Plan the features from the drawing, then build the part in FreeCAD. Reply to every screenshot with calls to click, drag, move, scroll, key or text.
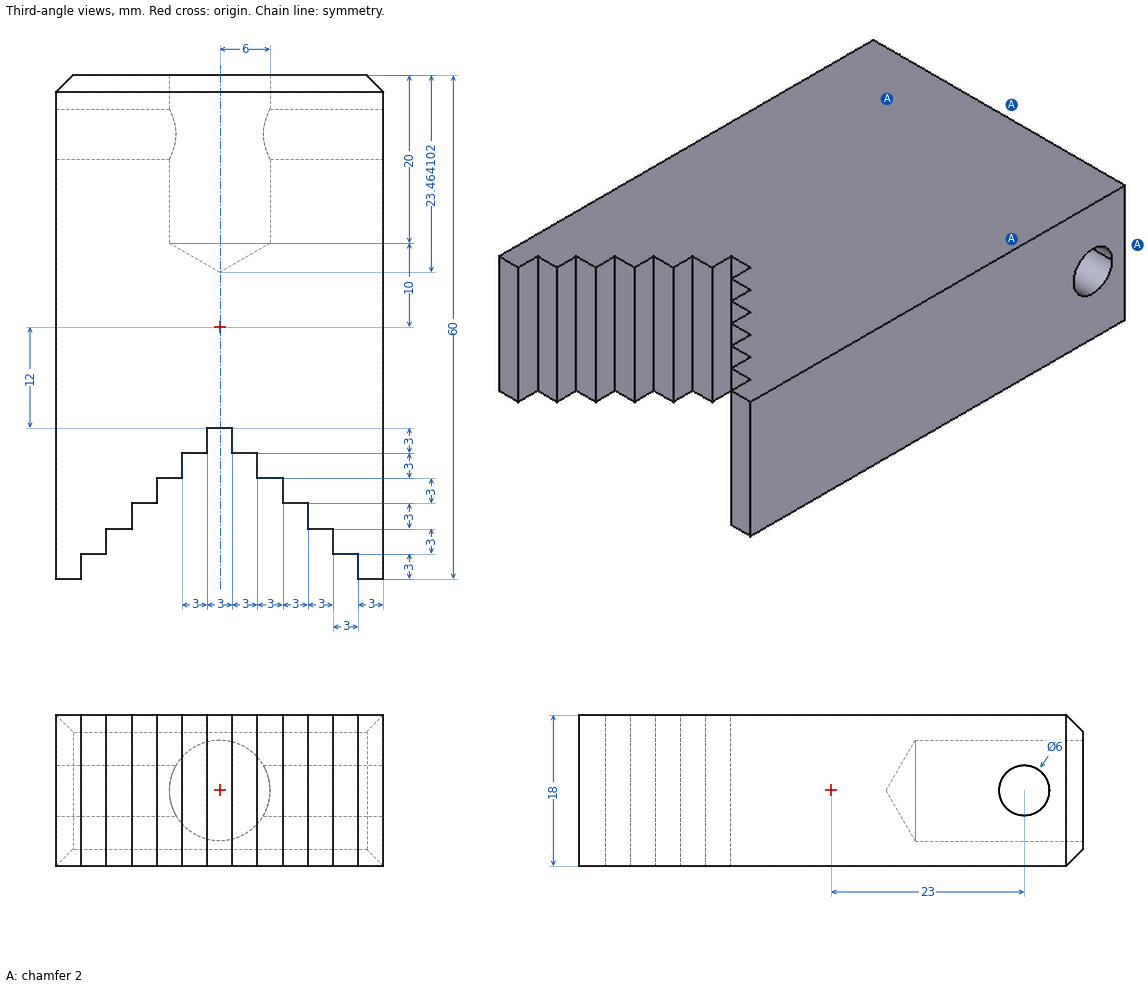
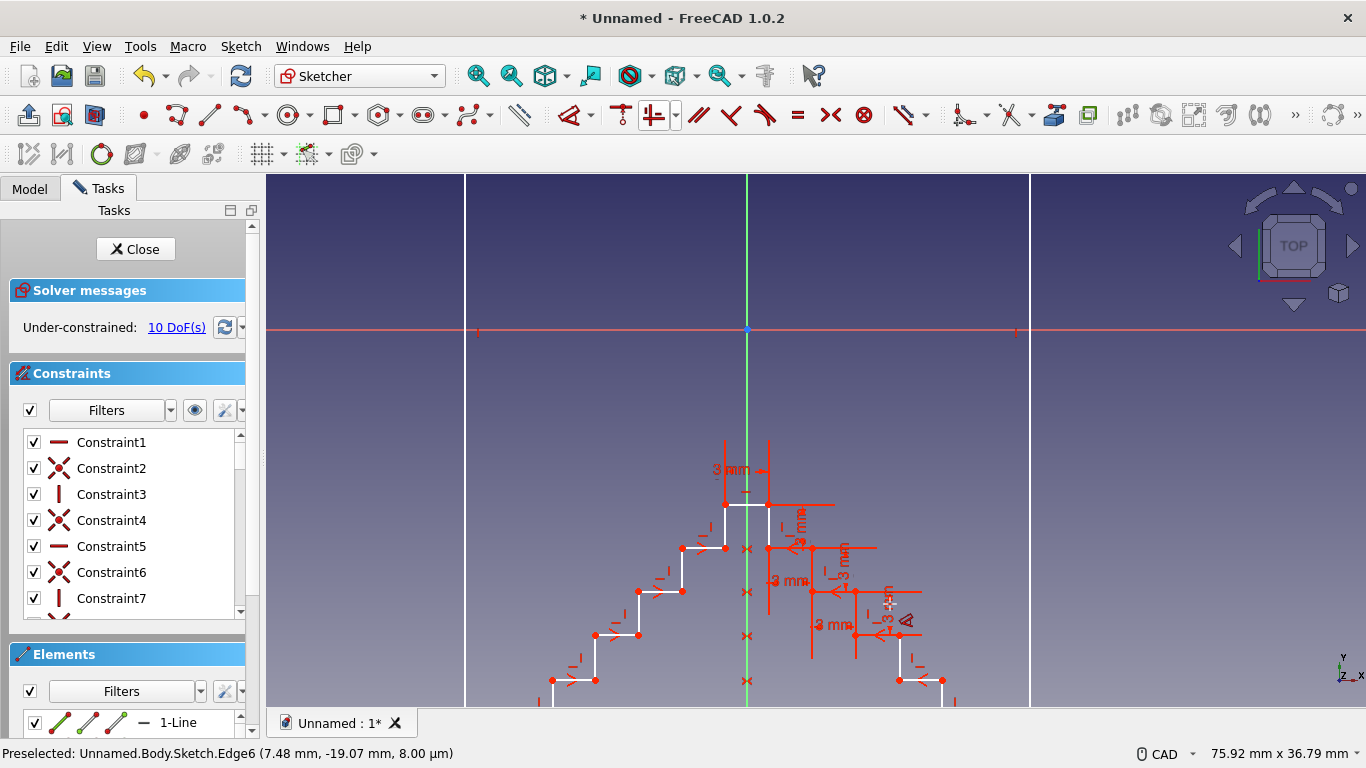
click(869, 635)
click(878, 669)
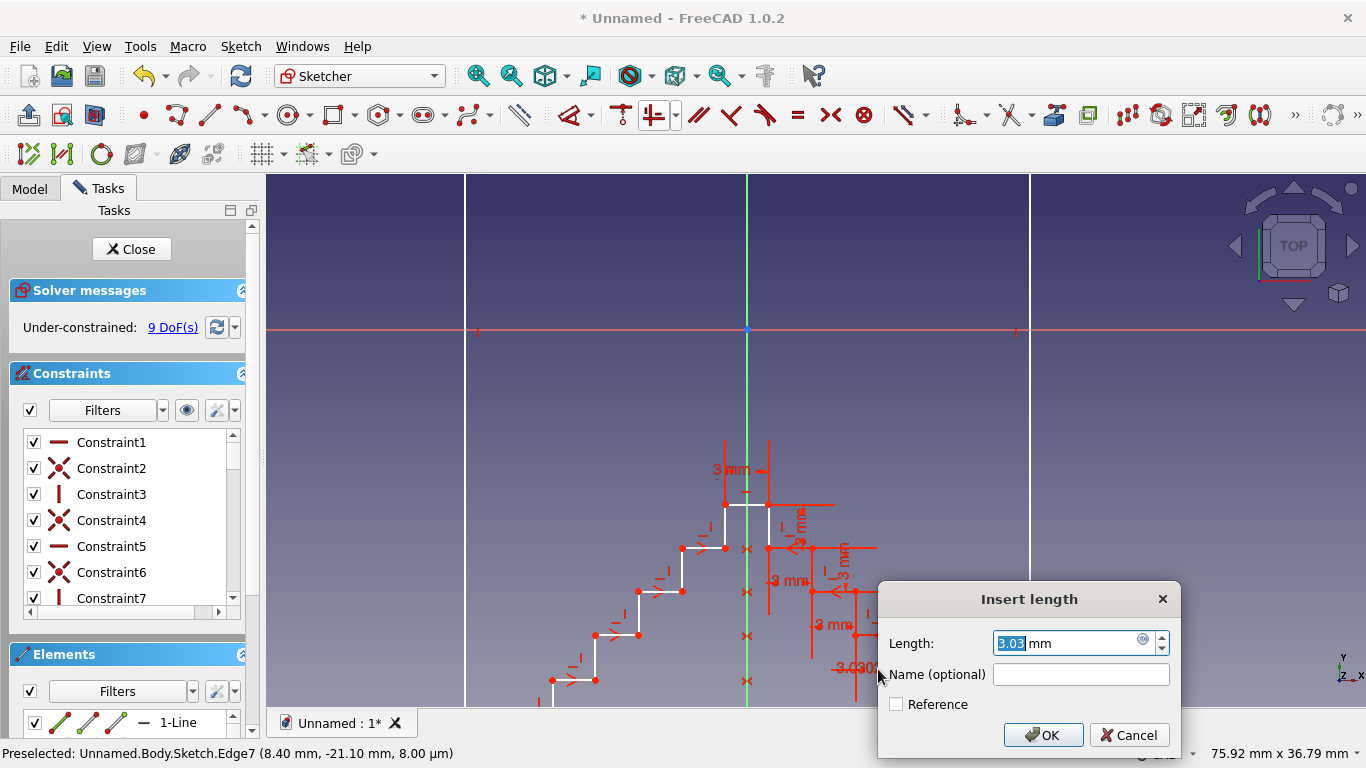
text(3)
key(Return)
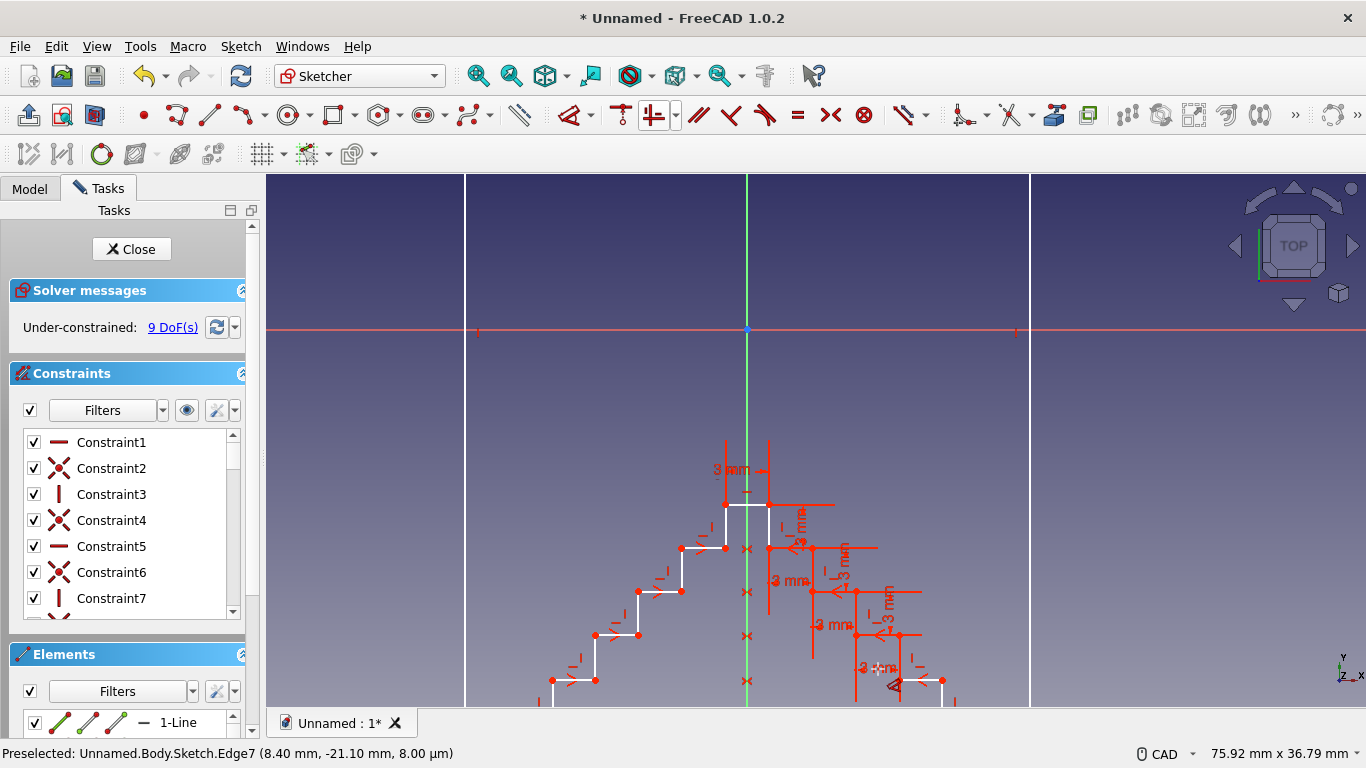
click(900, 649)
click(934, 647)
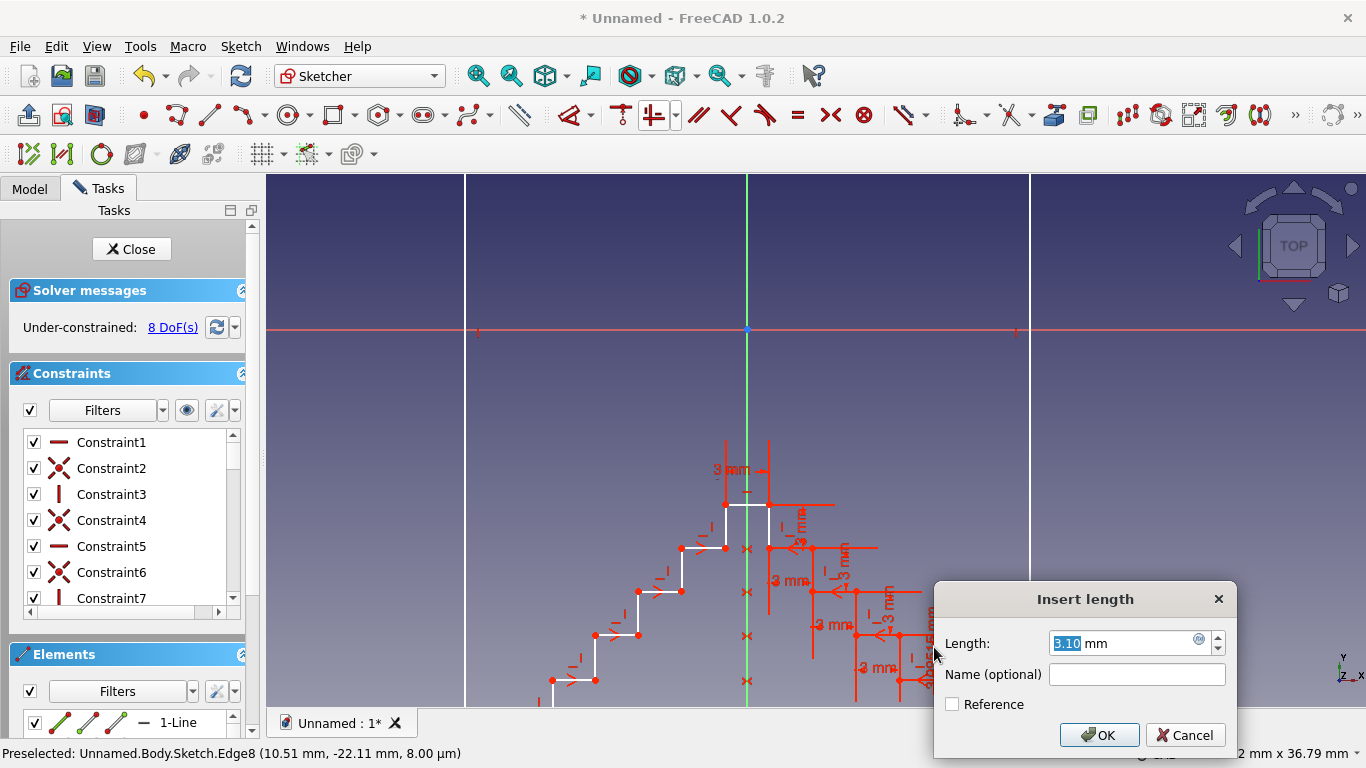
text(3)
key(Return)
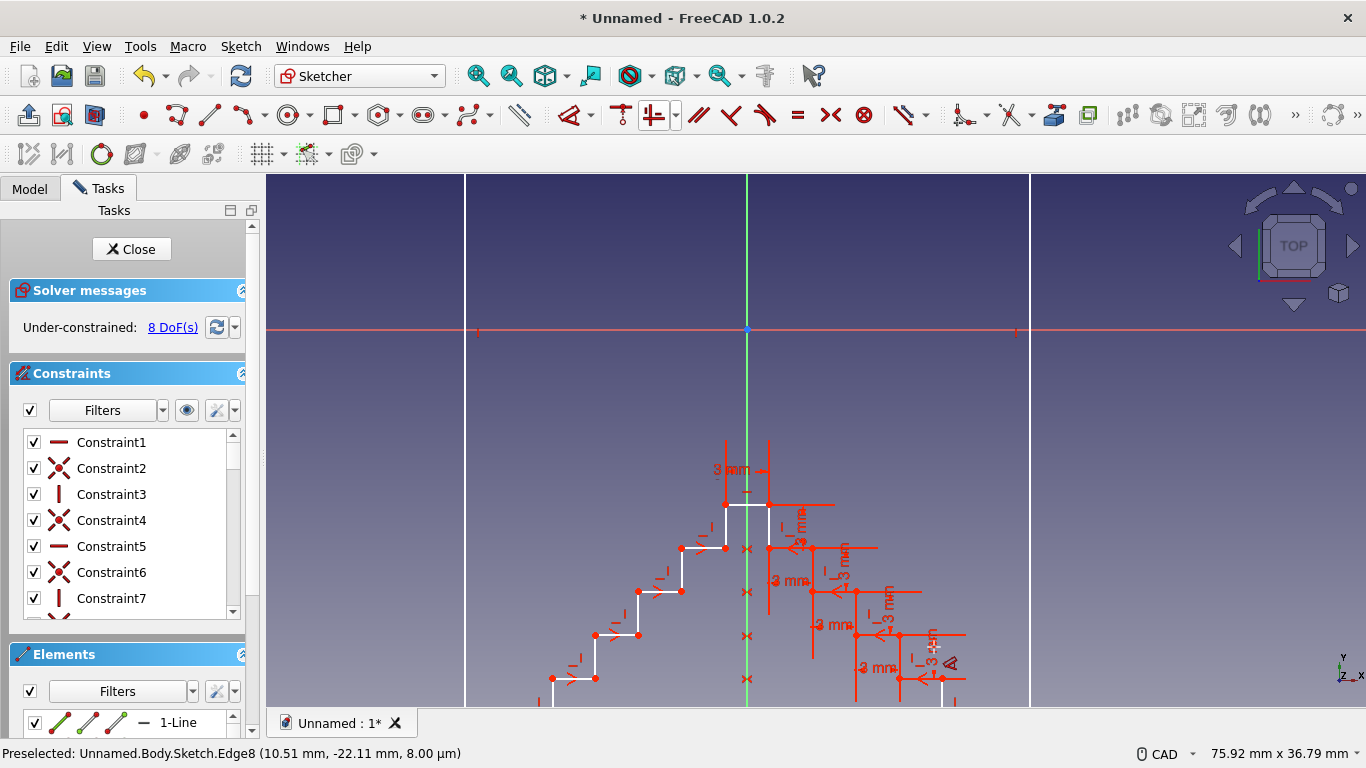
click(912, 679)
click(921, 573)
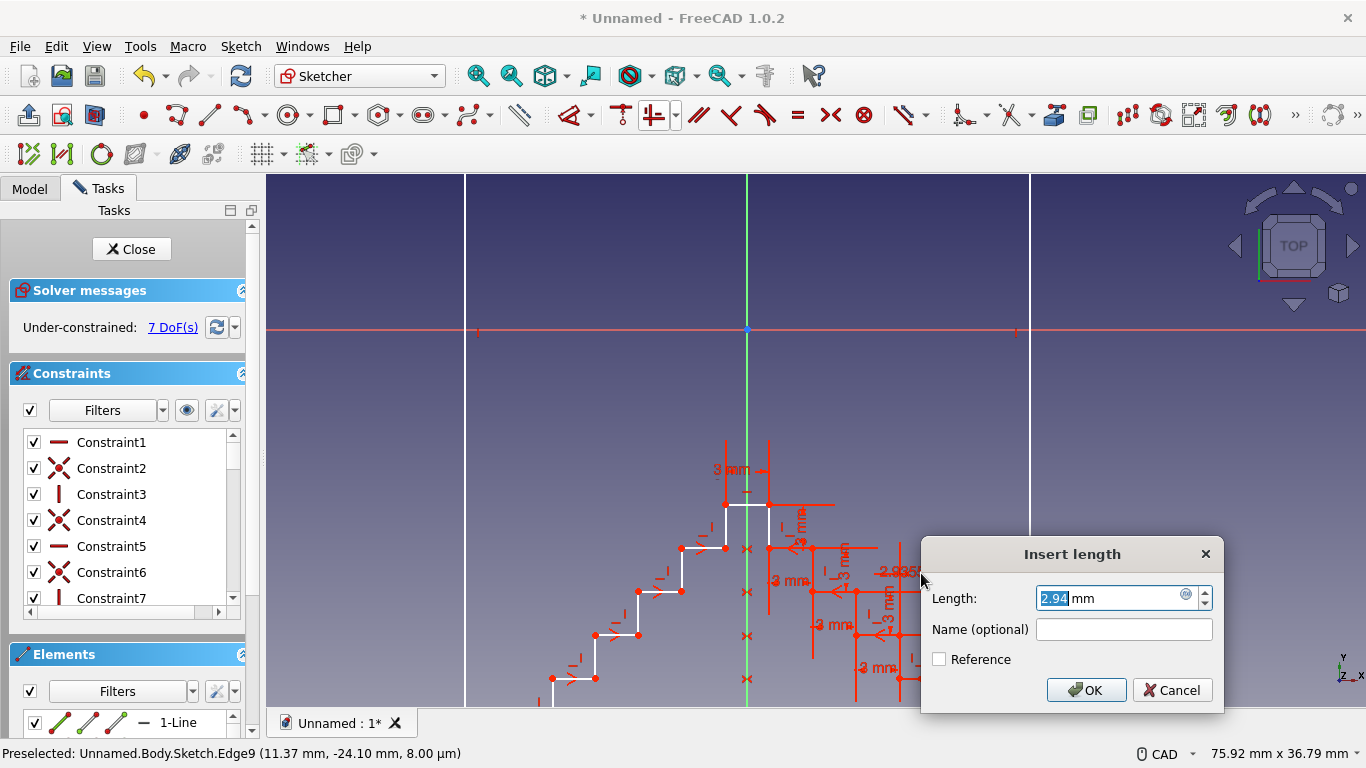
text(3)
key(Return)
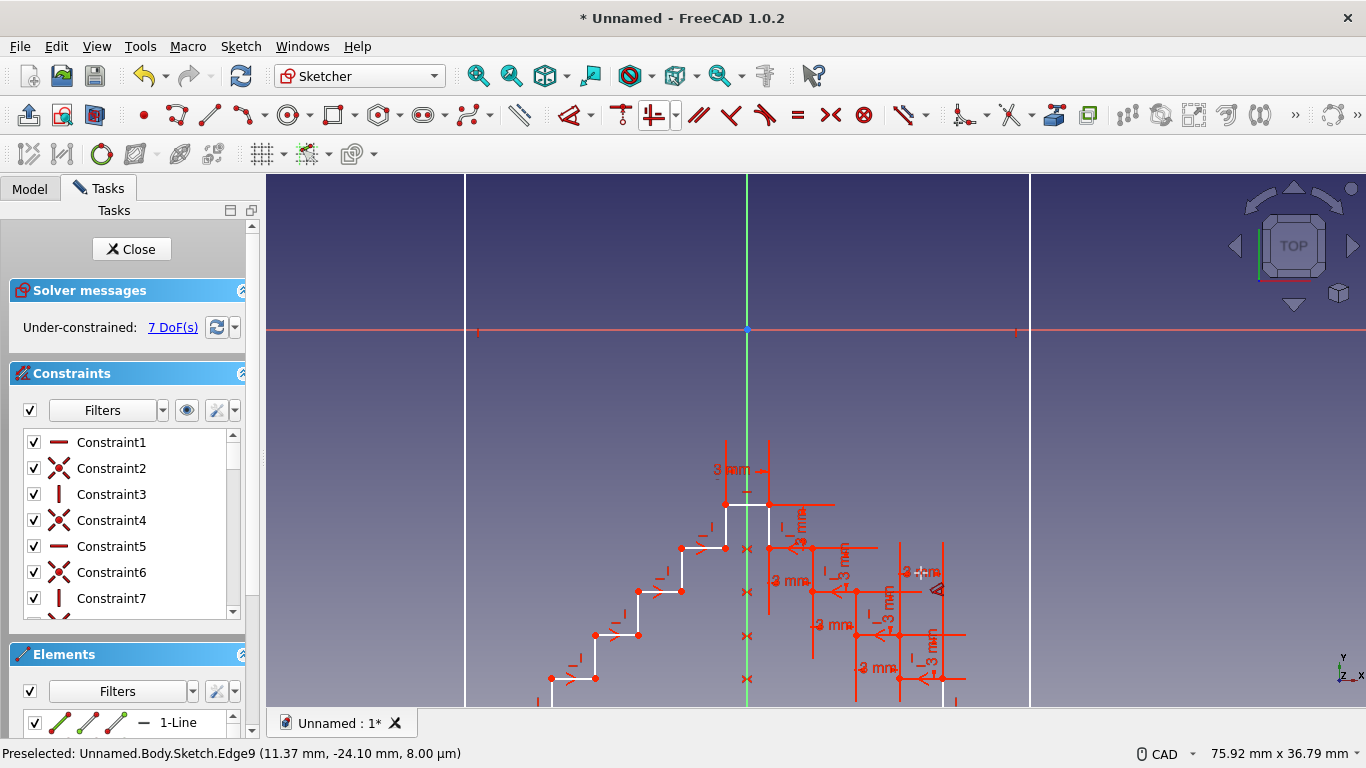
scroll(748, 505, down, 5)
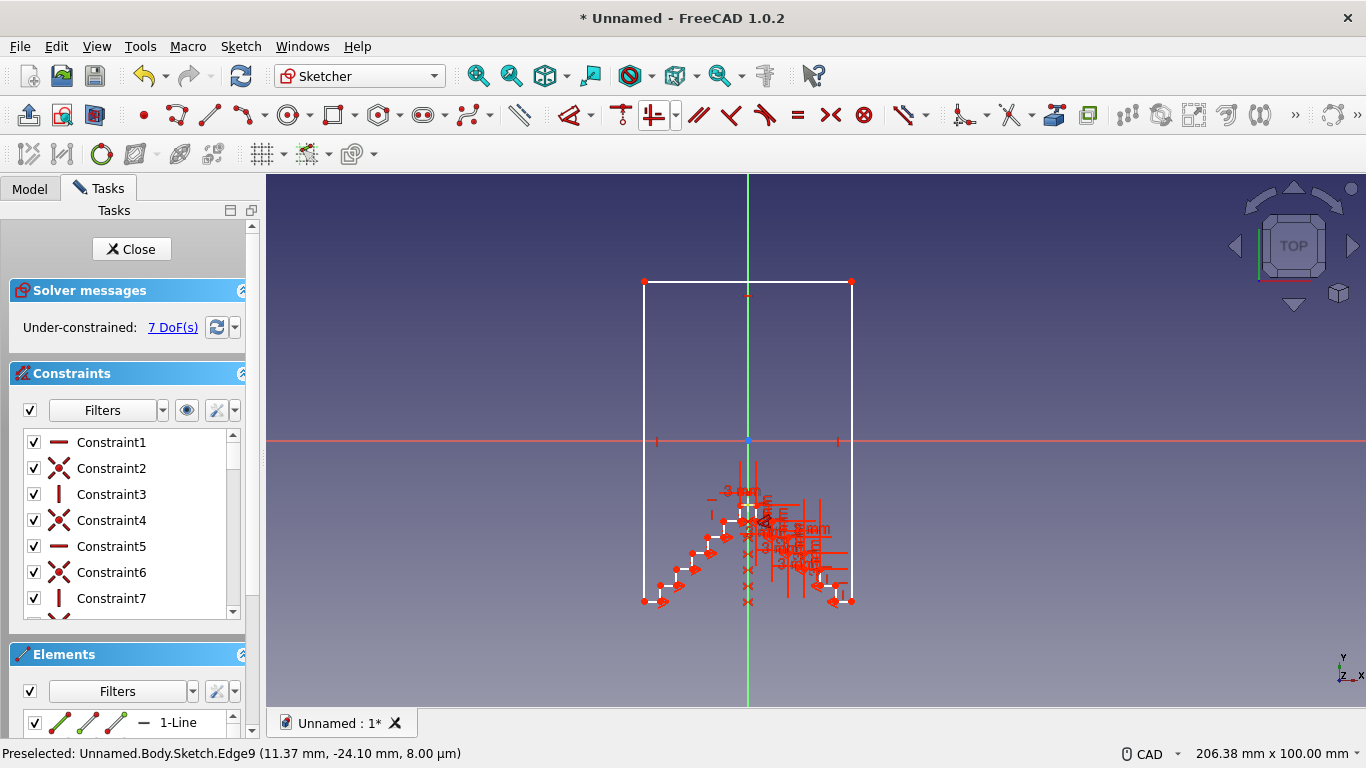
scroll(820, 574, up, 6)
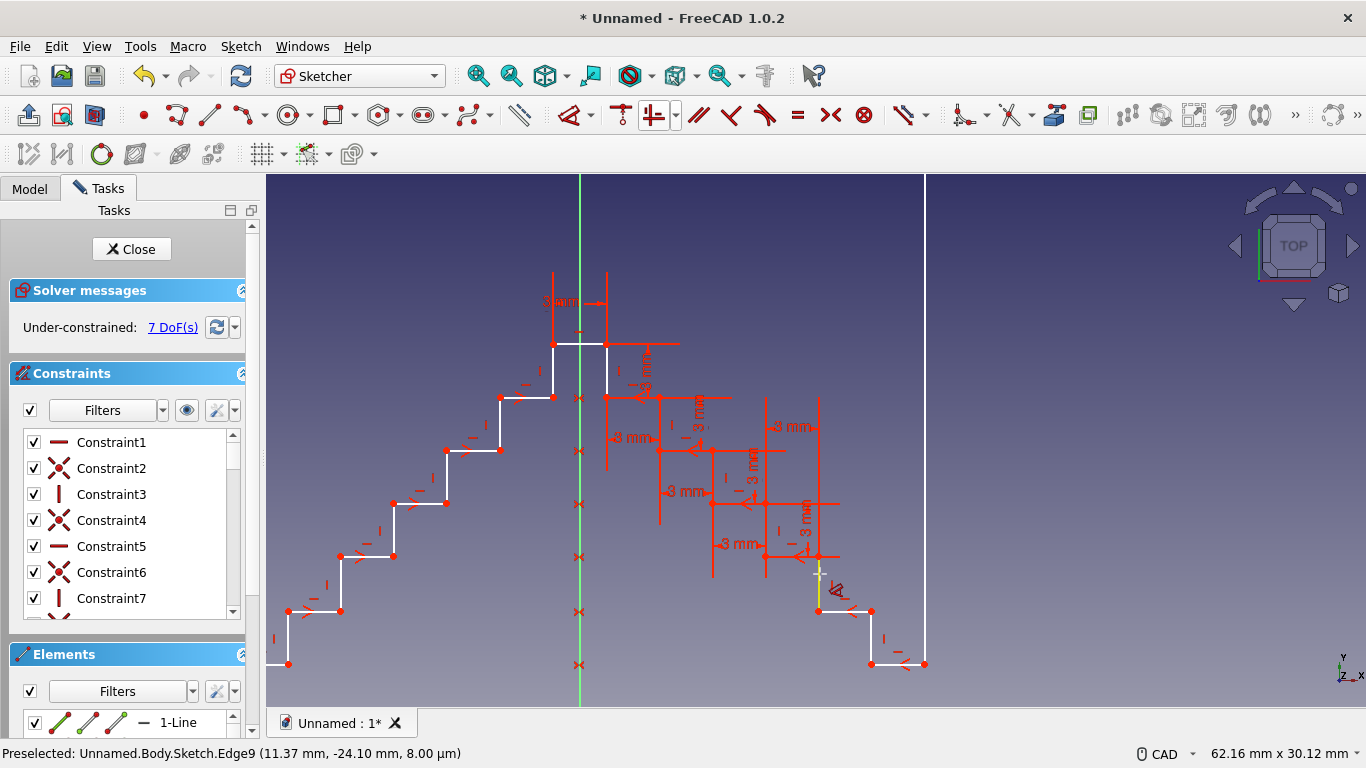
click(819, 573)
click(853, 584)